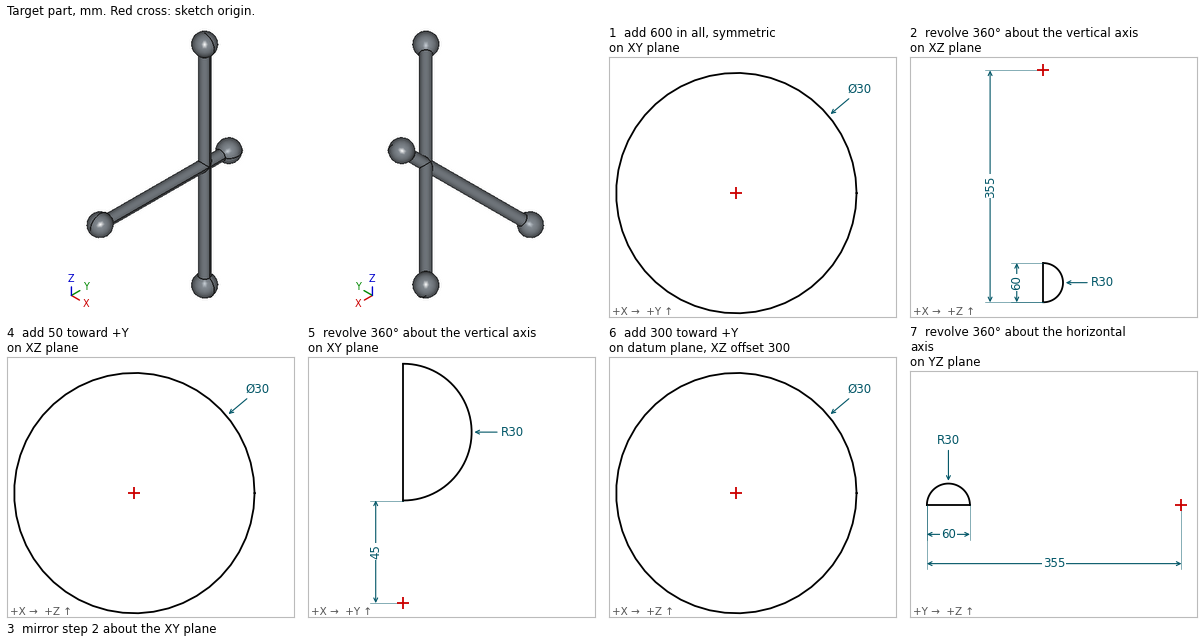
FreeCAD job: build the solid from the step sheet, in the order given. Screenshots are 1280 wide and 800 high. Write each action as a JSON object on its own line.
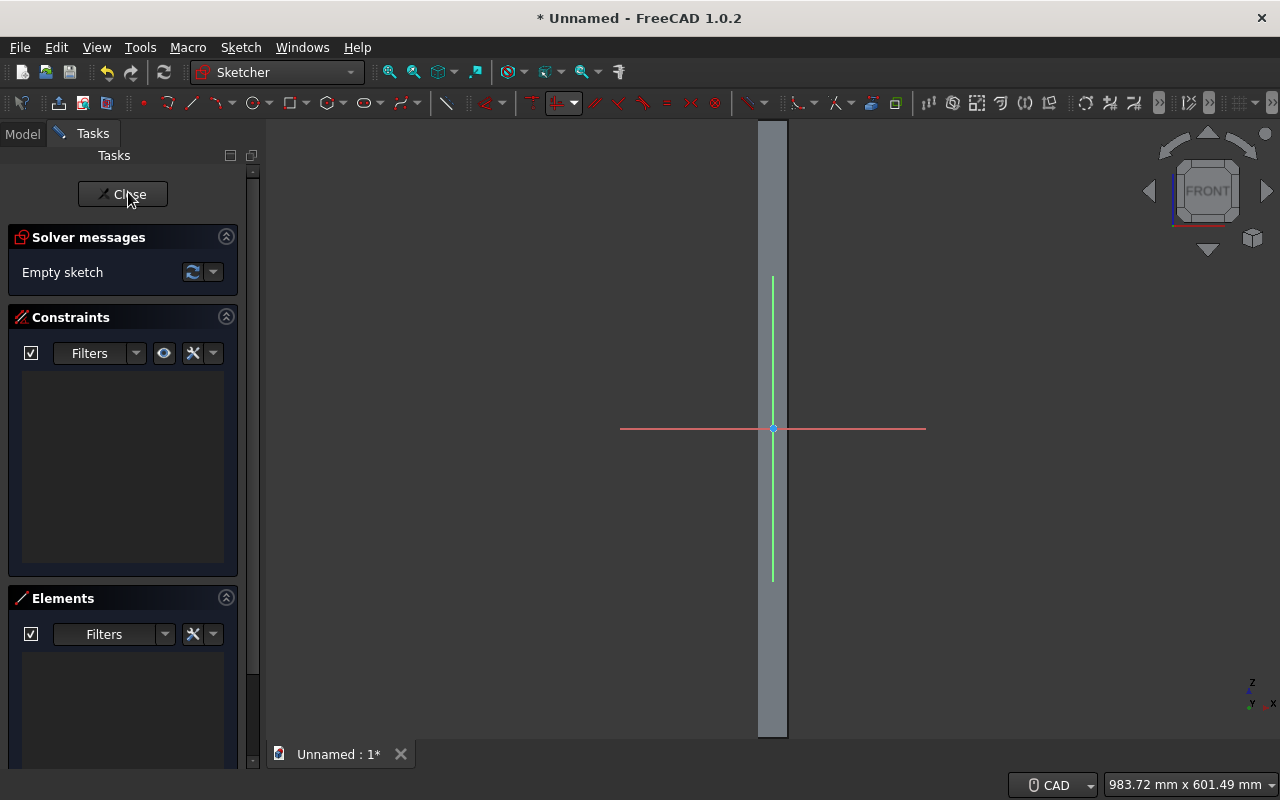
{"action": "scroll", "coordinate": [704, 429], "scroll_direction": "down", "scroll_amount": 5}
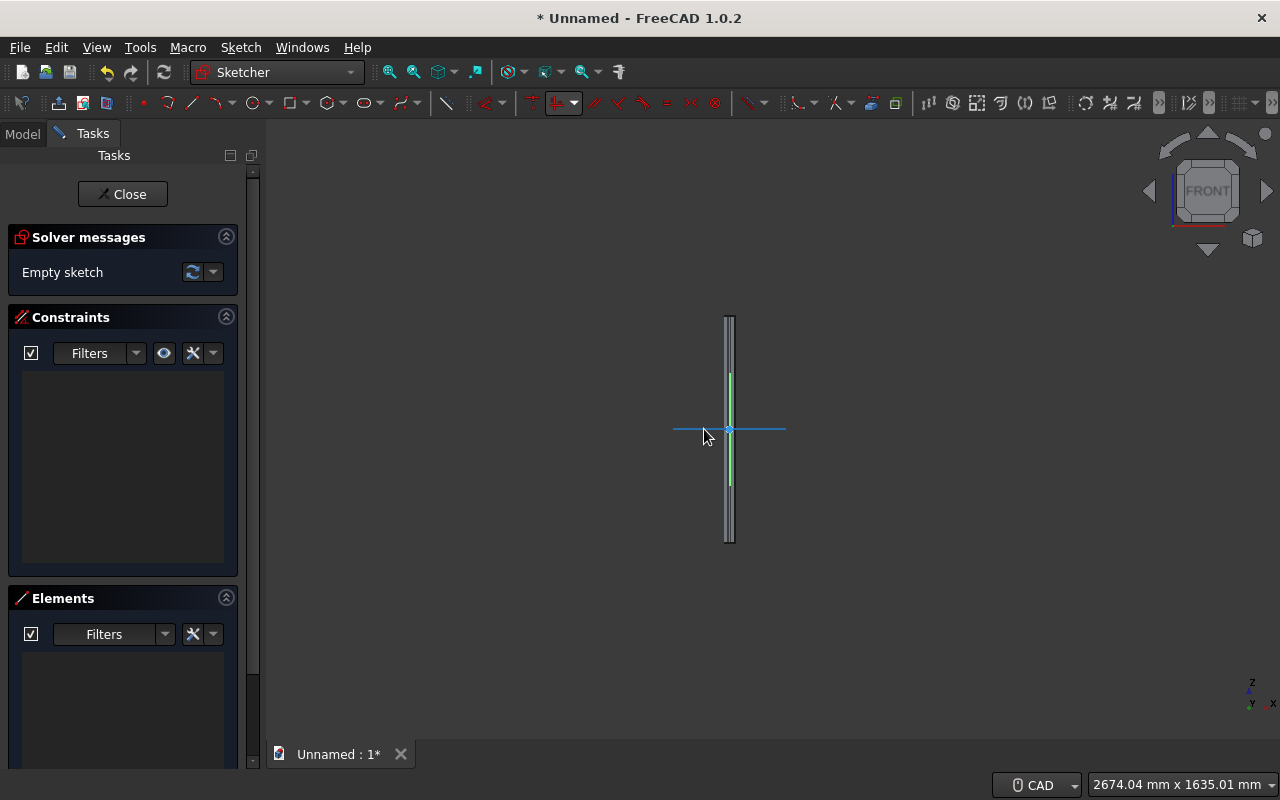
{"action": "scroll", "coordinate": [737, 561], "scroll_direction": "up", "scroll_amount": 14}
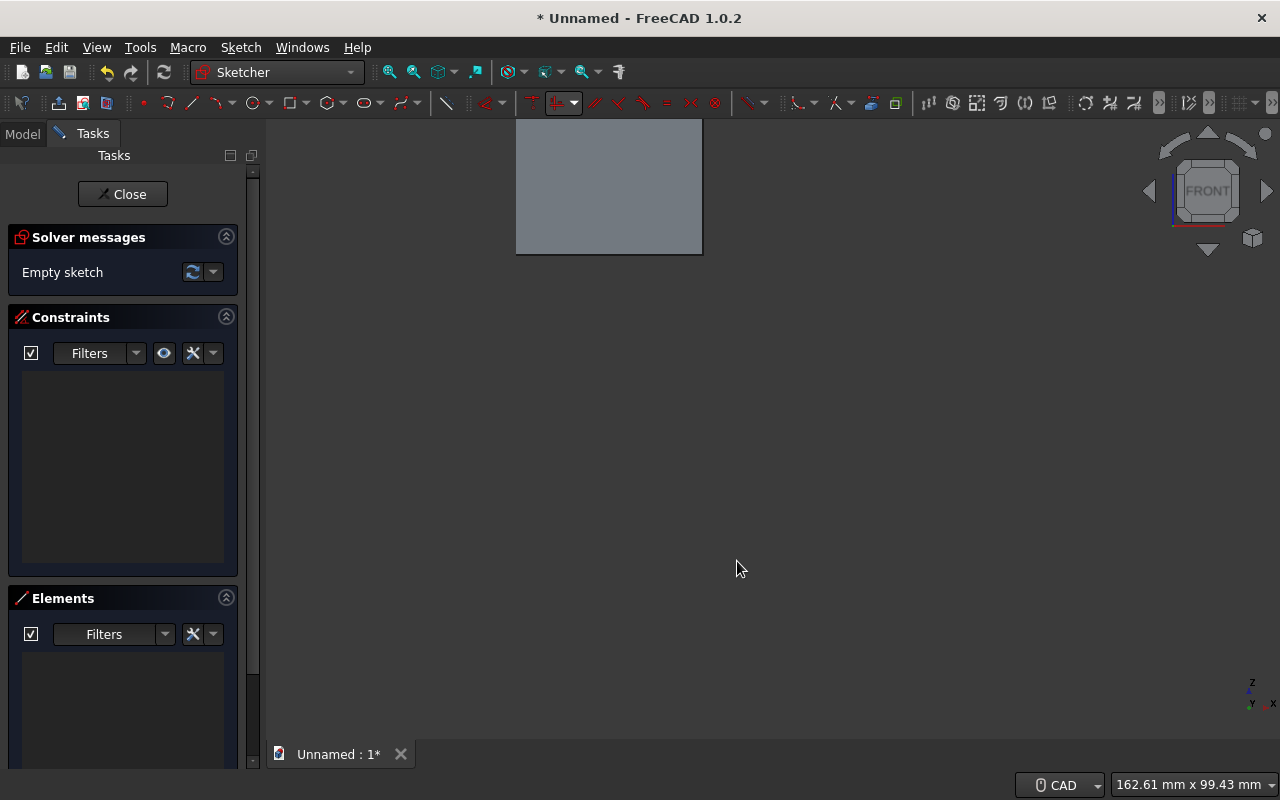
{"action": "left_click", "coordinate": [192, 104]}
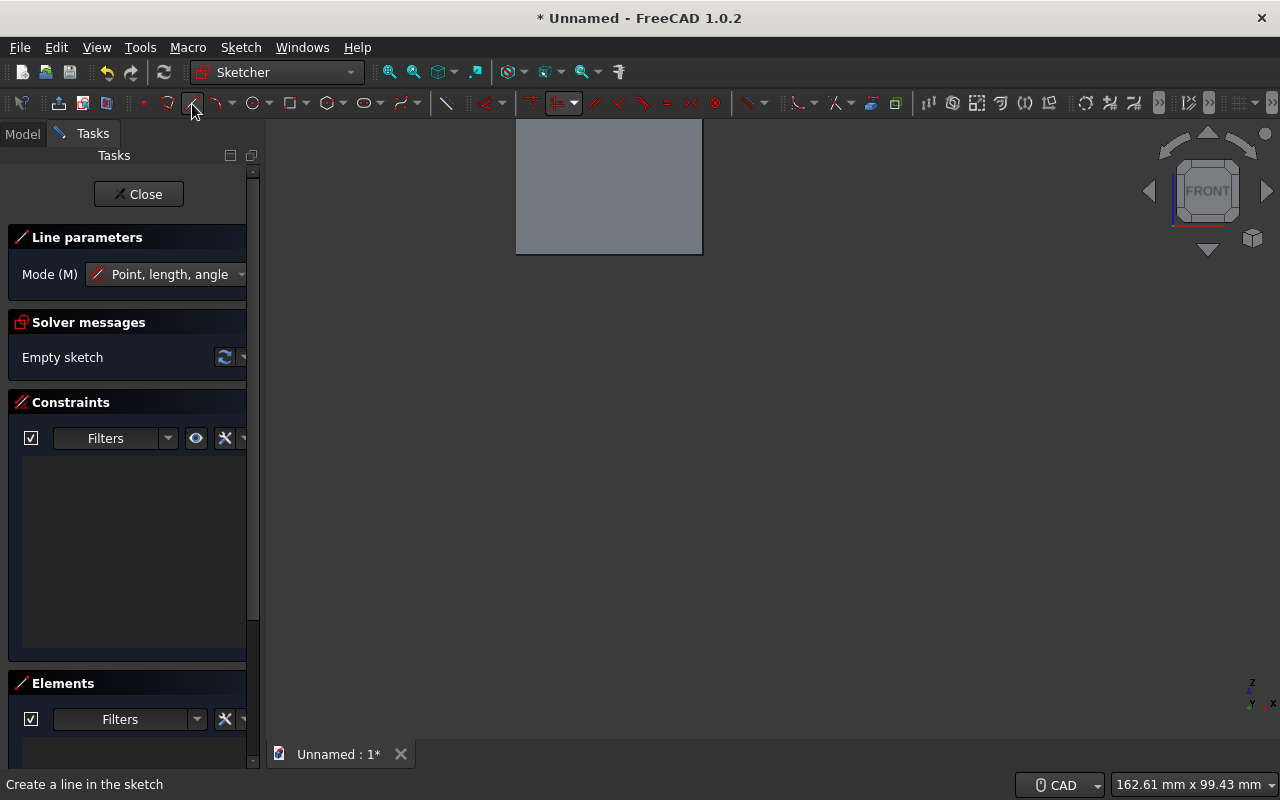
{"action": "left_click", "coordinate": [609, 598]}
{"action": "left_click", "coordinate": [618, 224]}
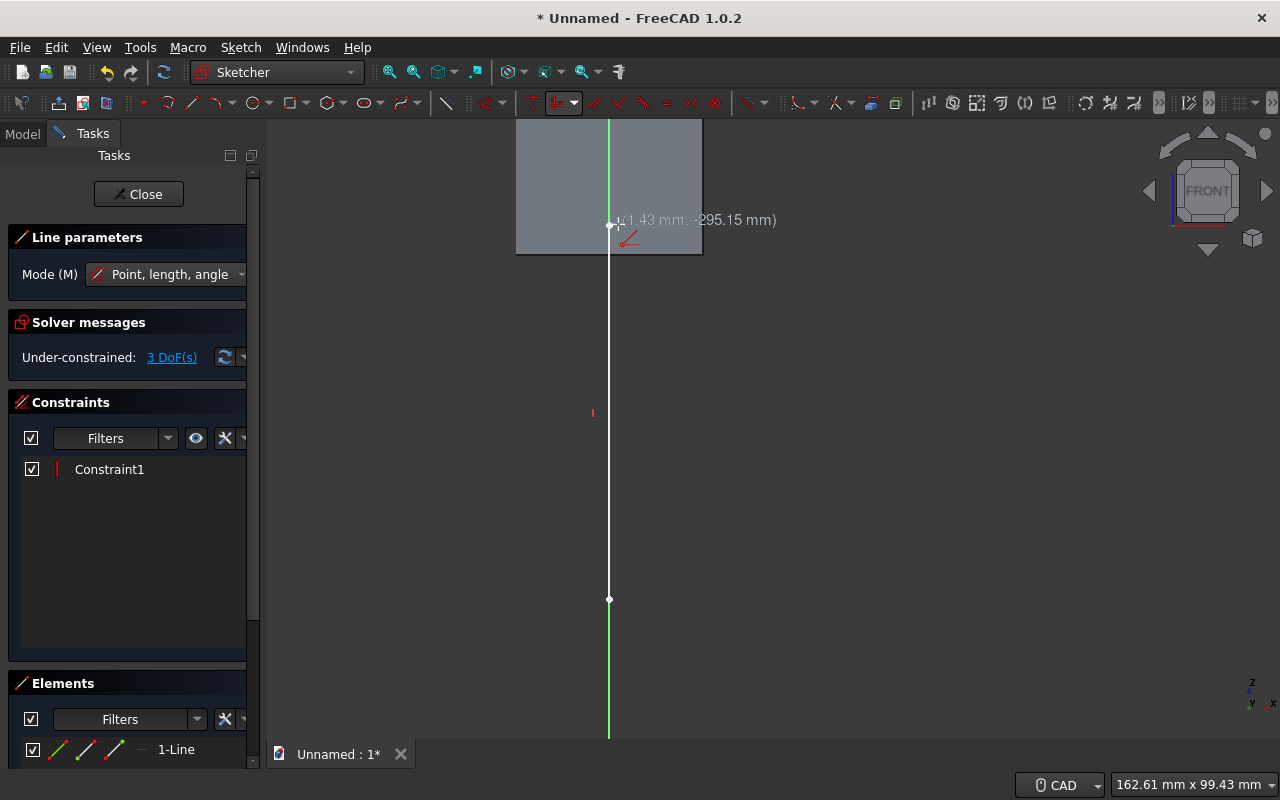
{"action": "left_click", "coordinate": [216, 104]}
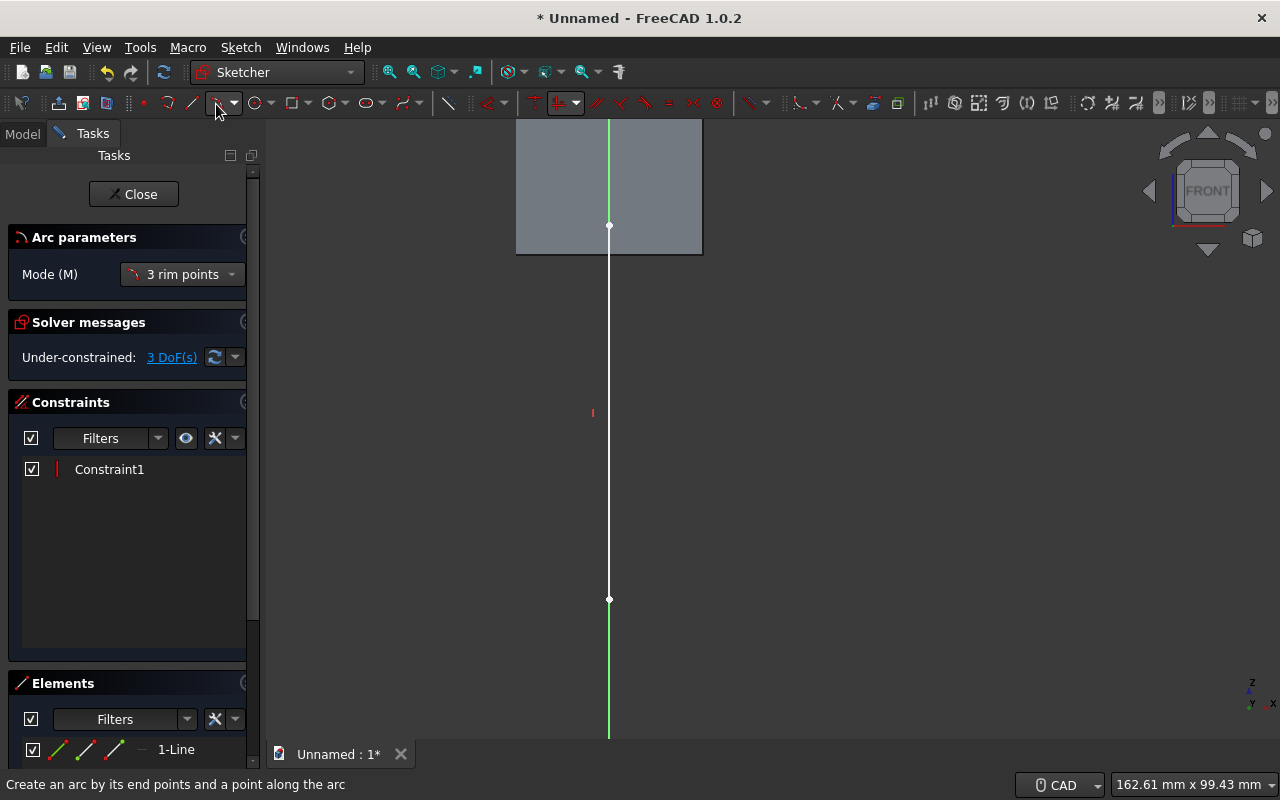
{"action": "left_click", "coordinate": [618, 224]}
{"action": "left_click", "coordinate": [609, 599]}
{"action": "left_click", "coordinate": [796, 411]}
{"action": "key", "text": "Escape"}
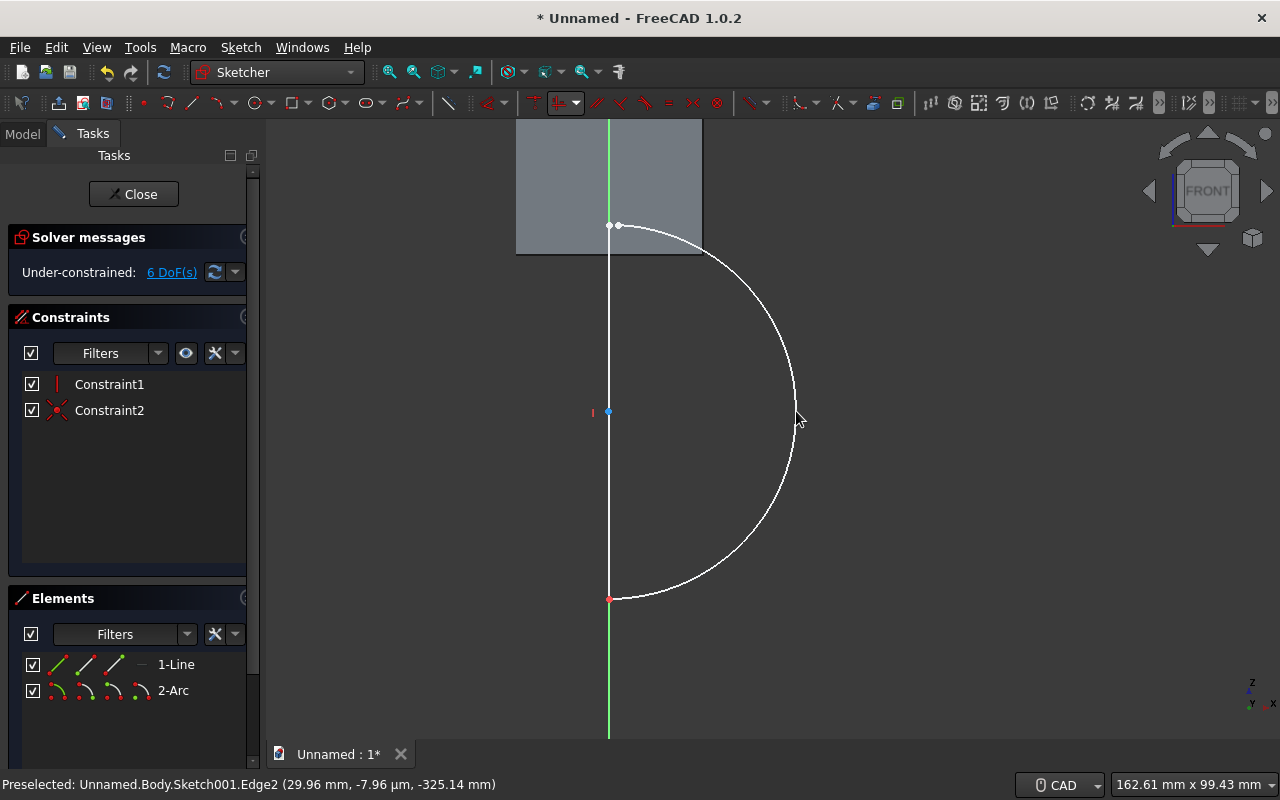
{"action": "left_click", "coordinate": [609, 412]}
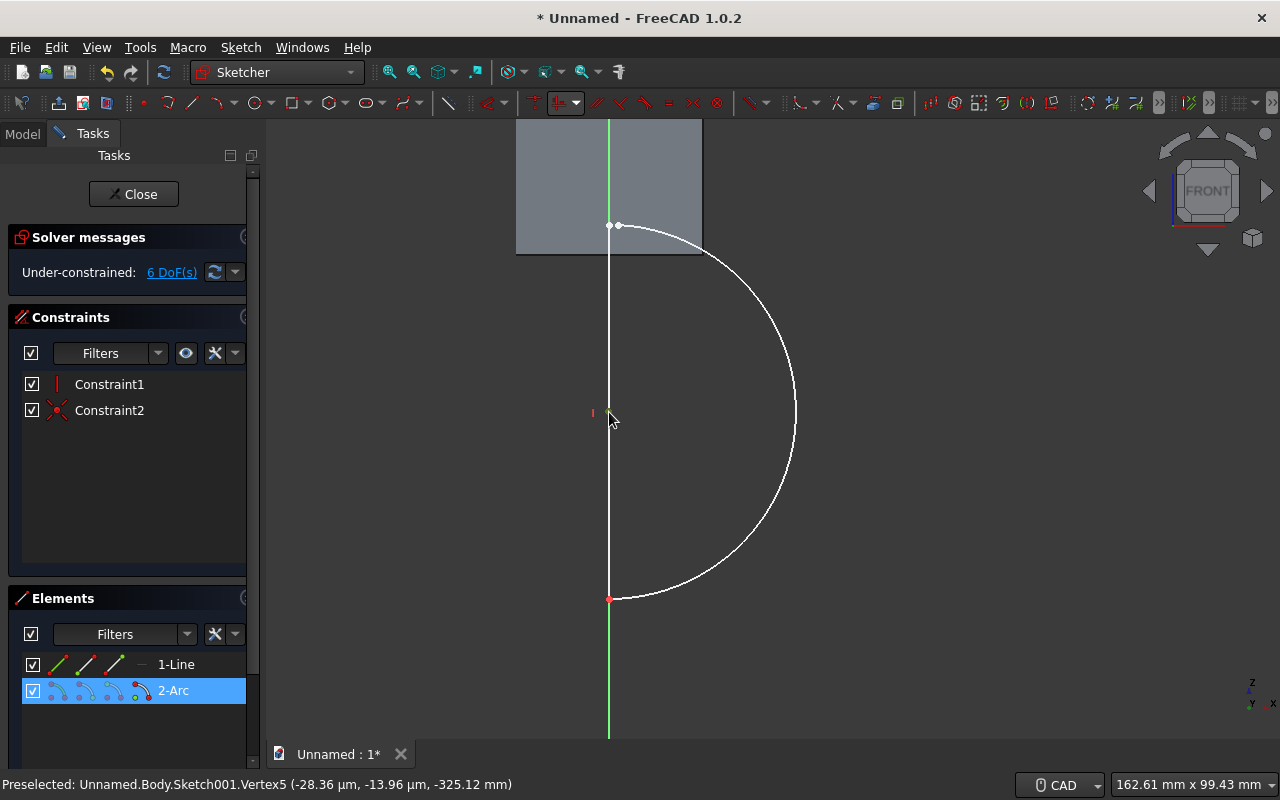
{"action": "left_click", "coordinate": [609, 671]}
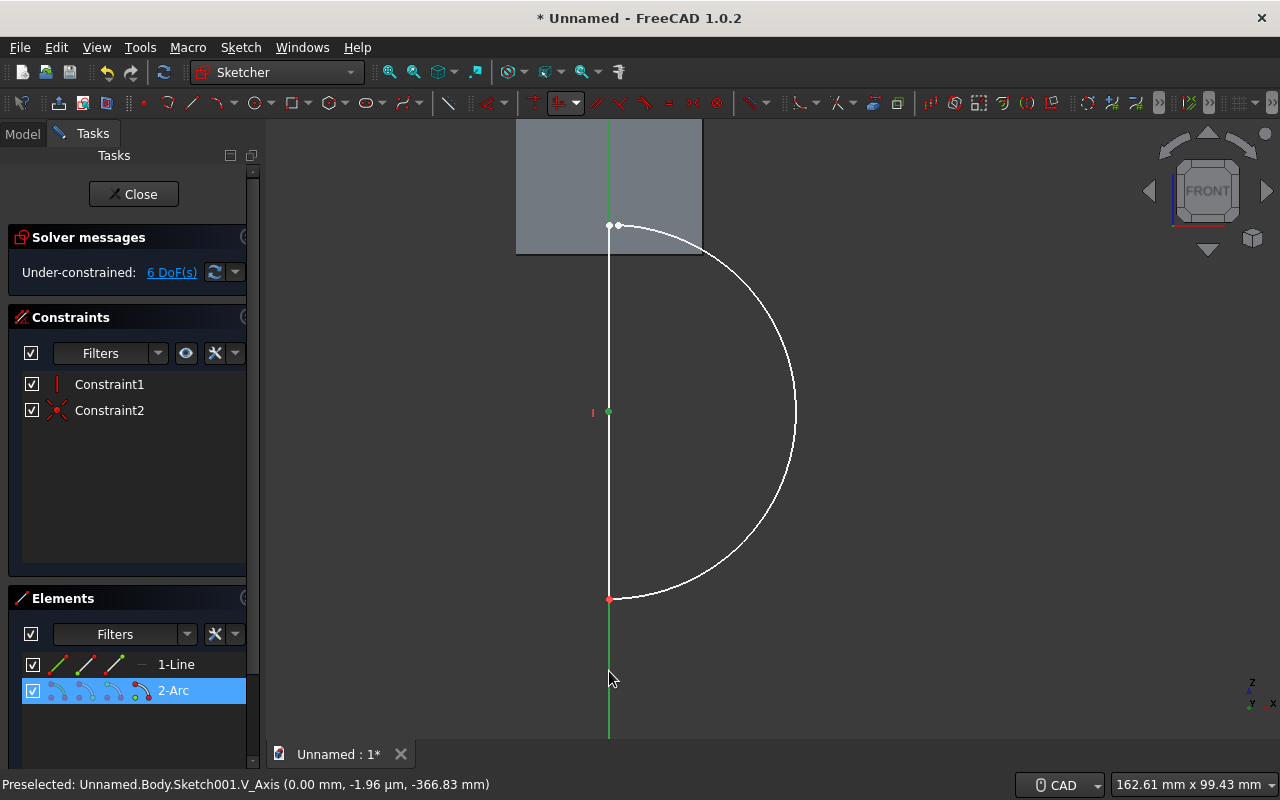
{"action": "left_click", "coordinate": [534, 104]}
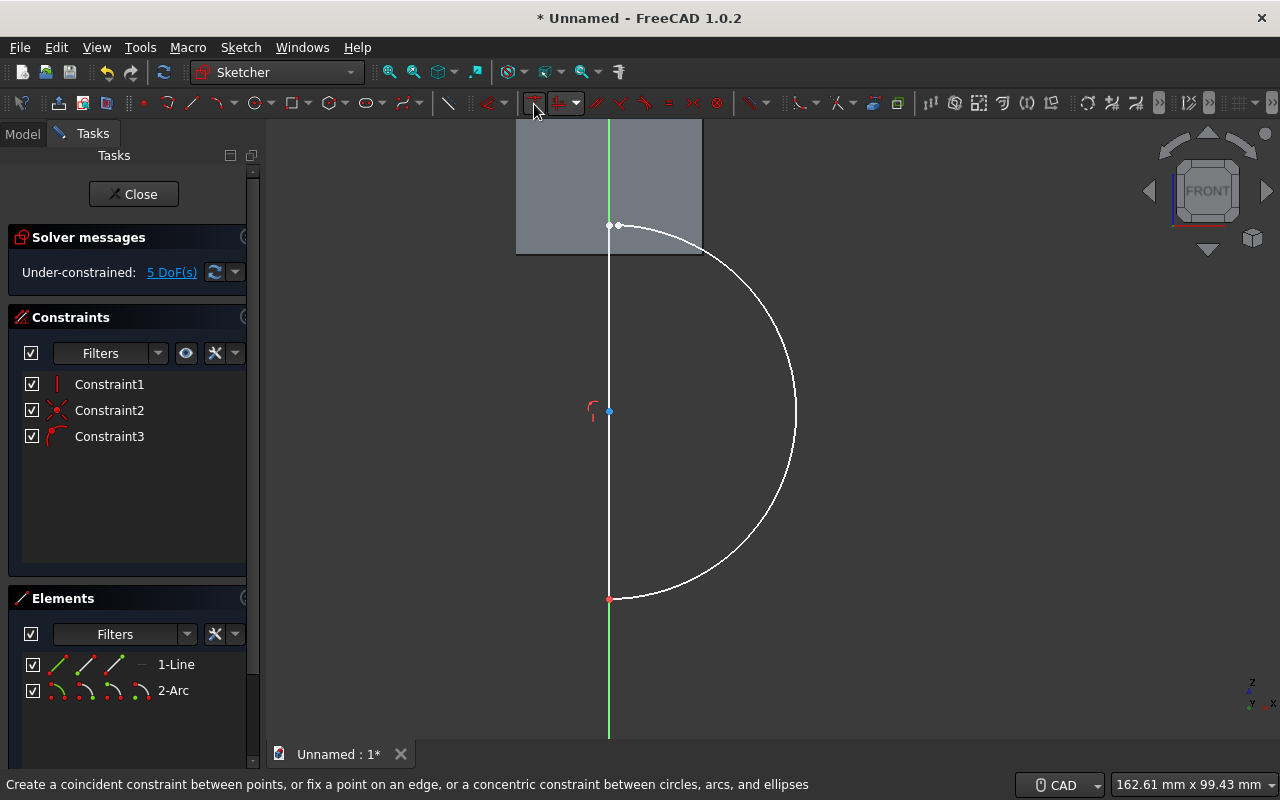
{"action": "left_click", "coordinate": [759, 524]}